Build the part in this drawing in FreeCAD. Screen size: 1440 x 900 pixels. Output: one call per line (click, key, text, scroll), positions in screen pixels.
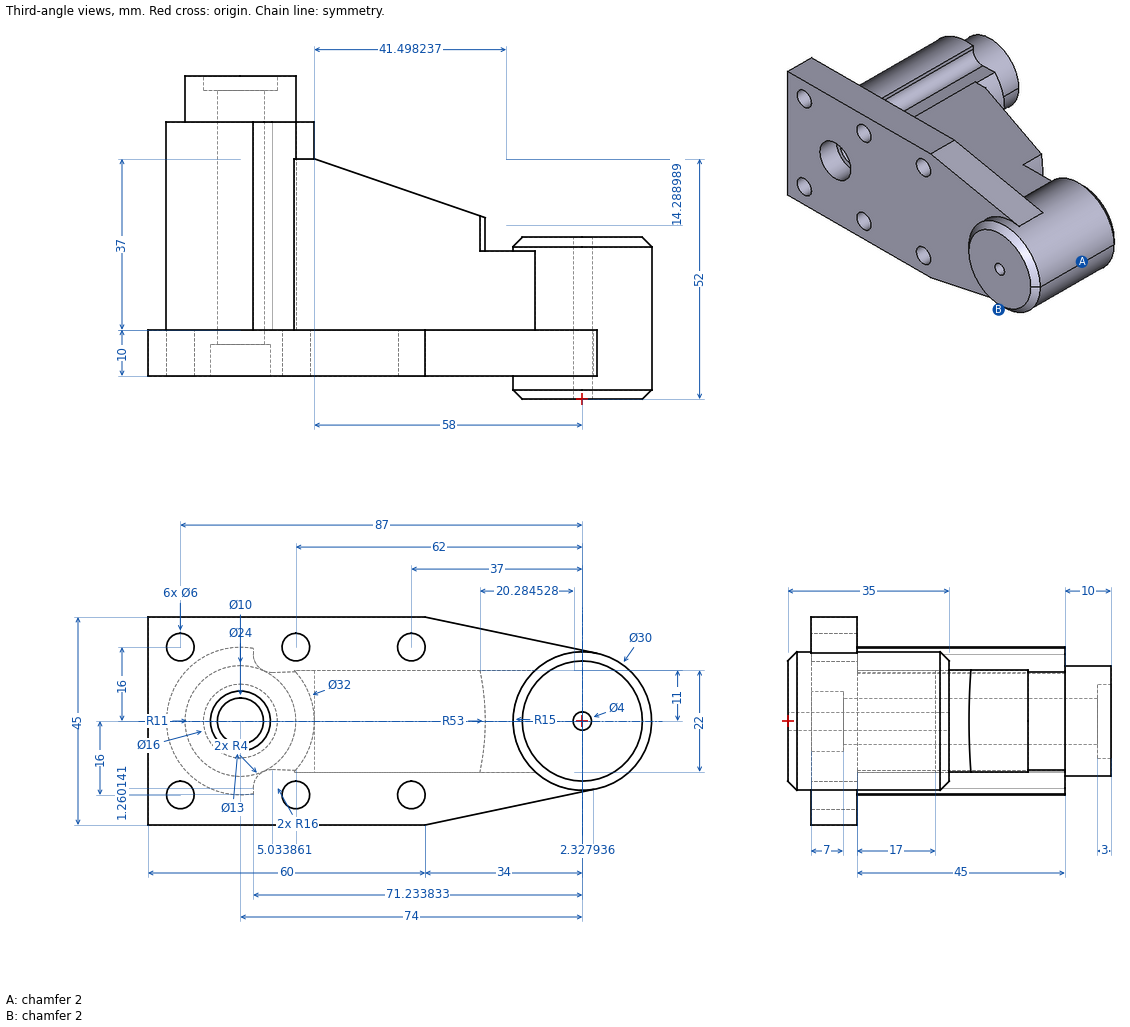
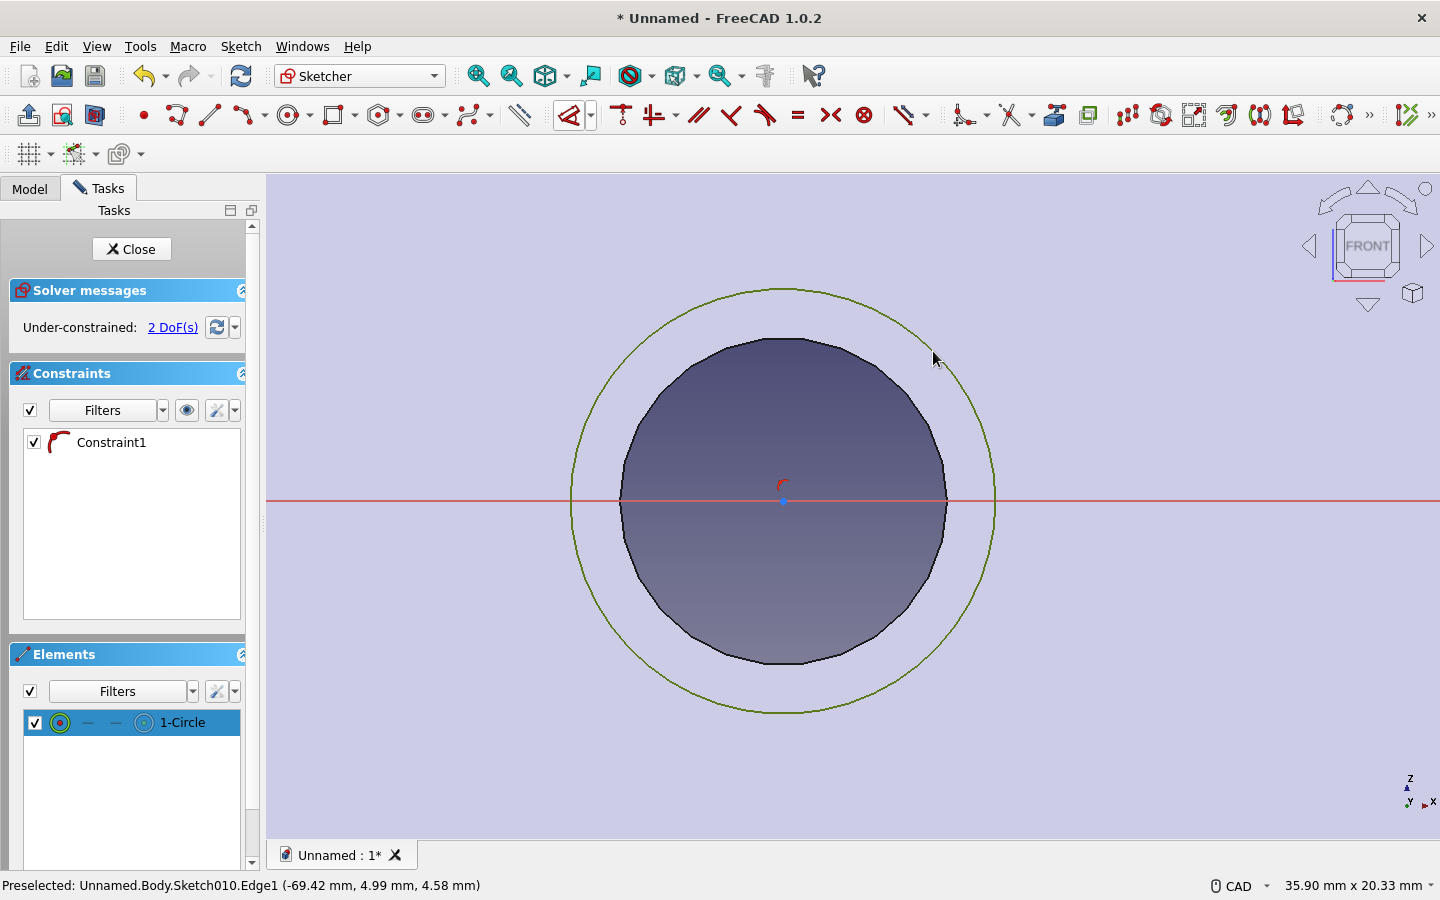
key(k)
key(o)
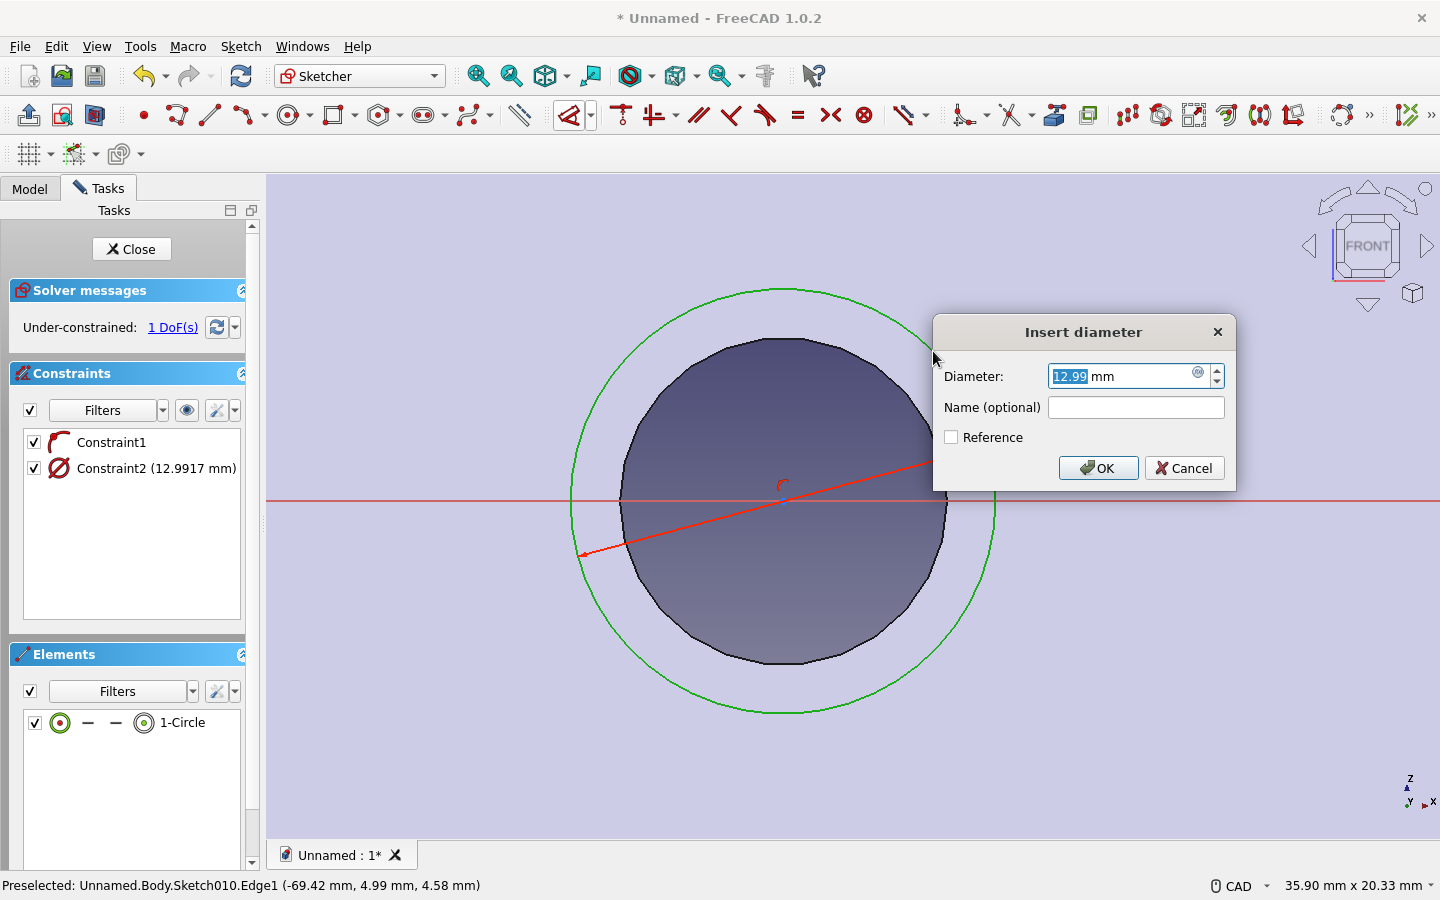
text(13)
key(Return)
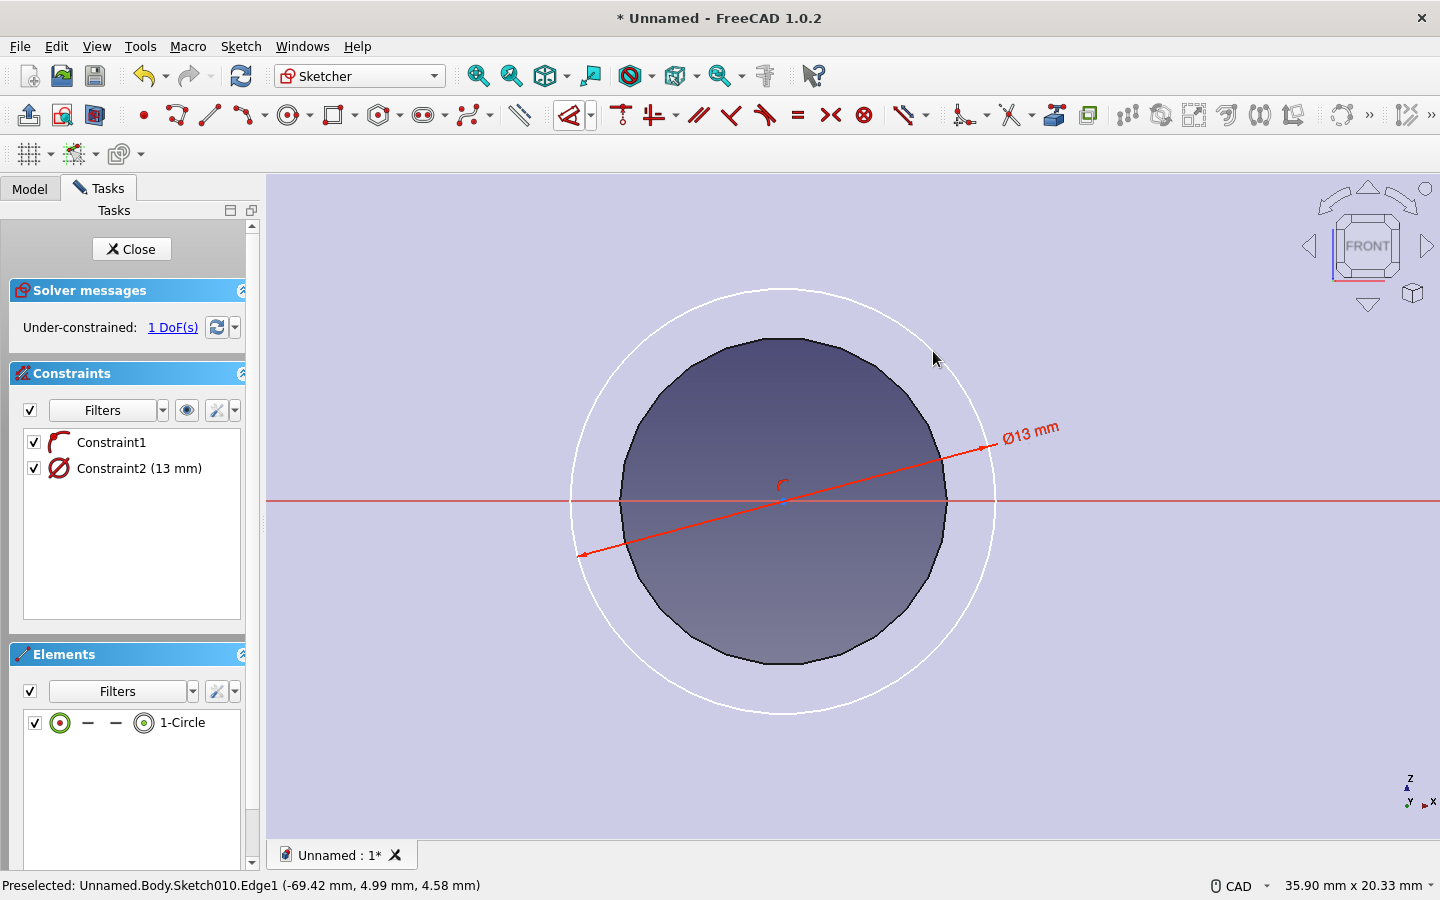
click(783, 501)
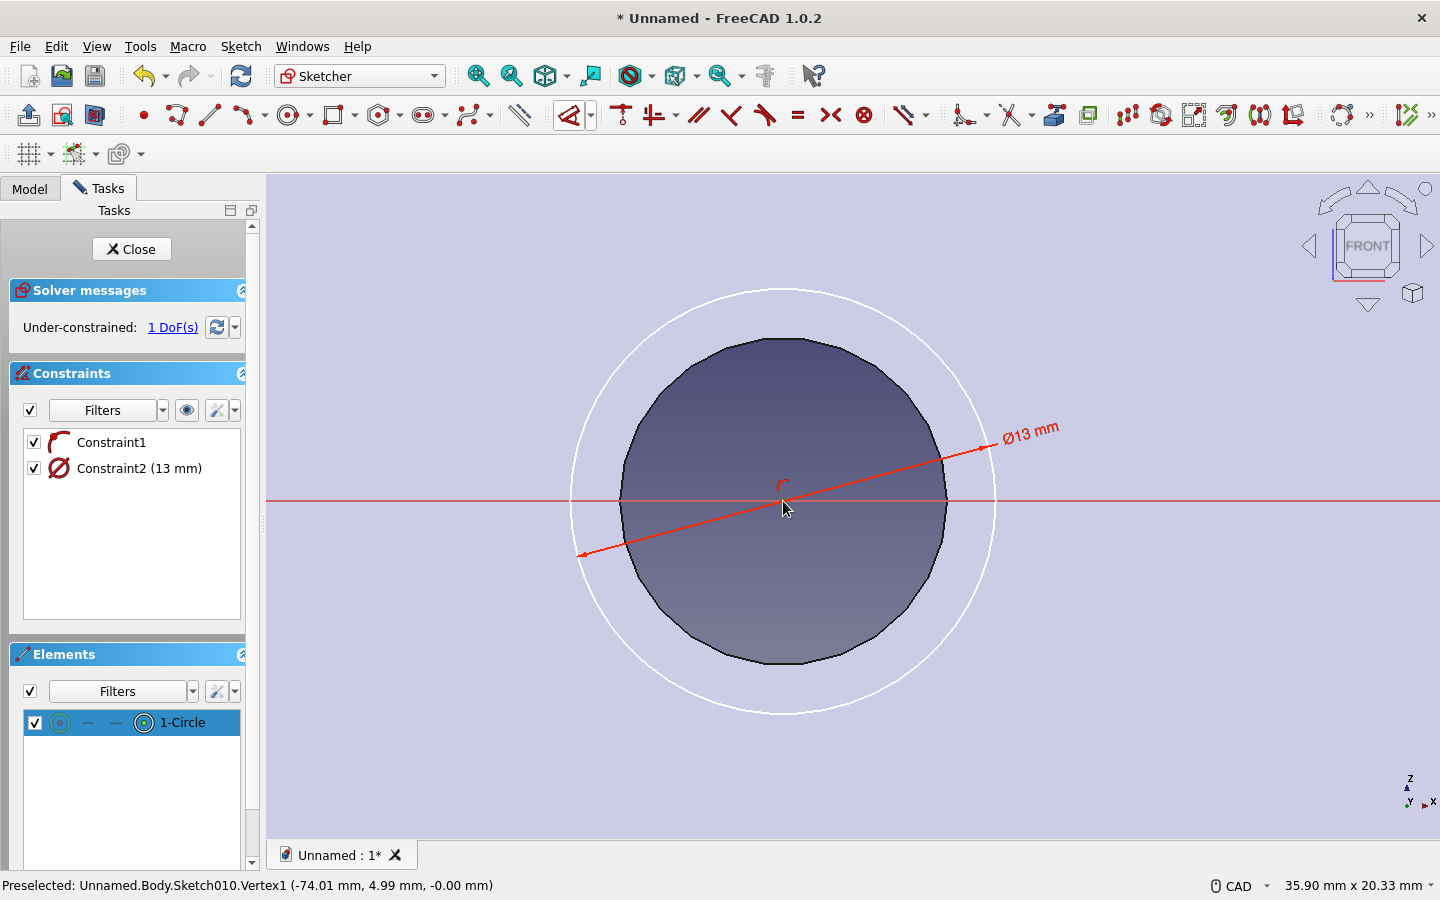
click(590, 116)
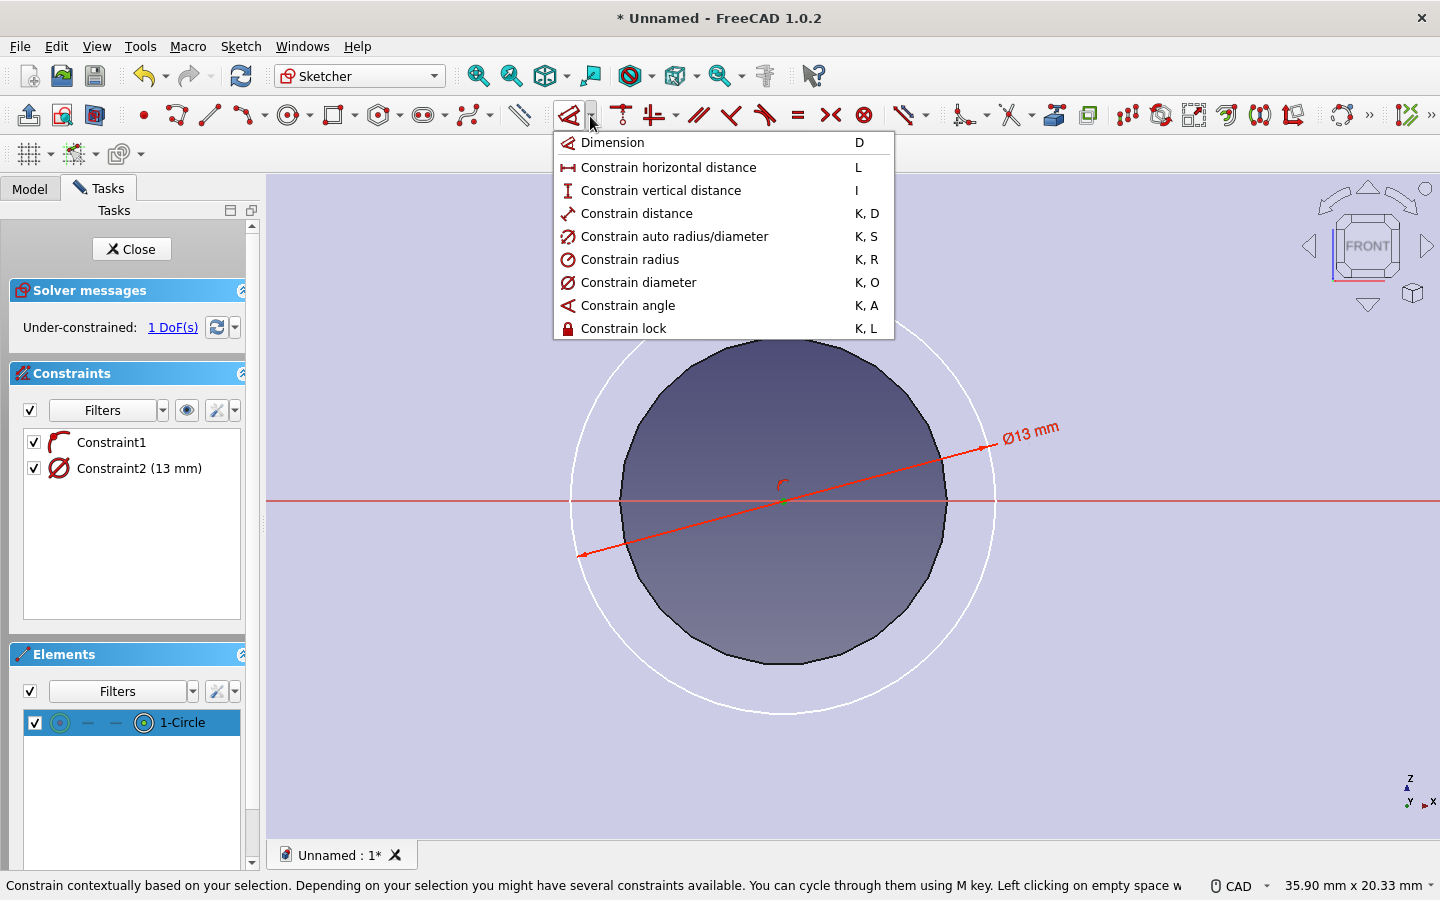
click(724, 168)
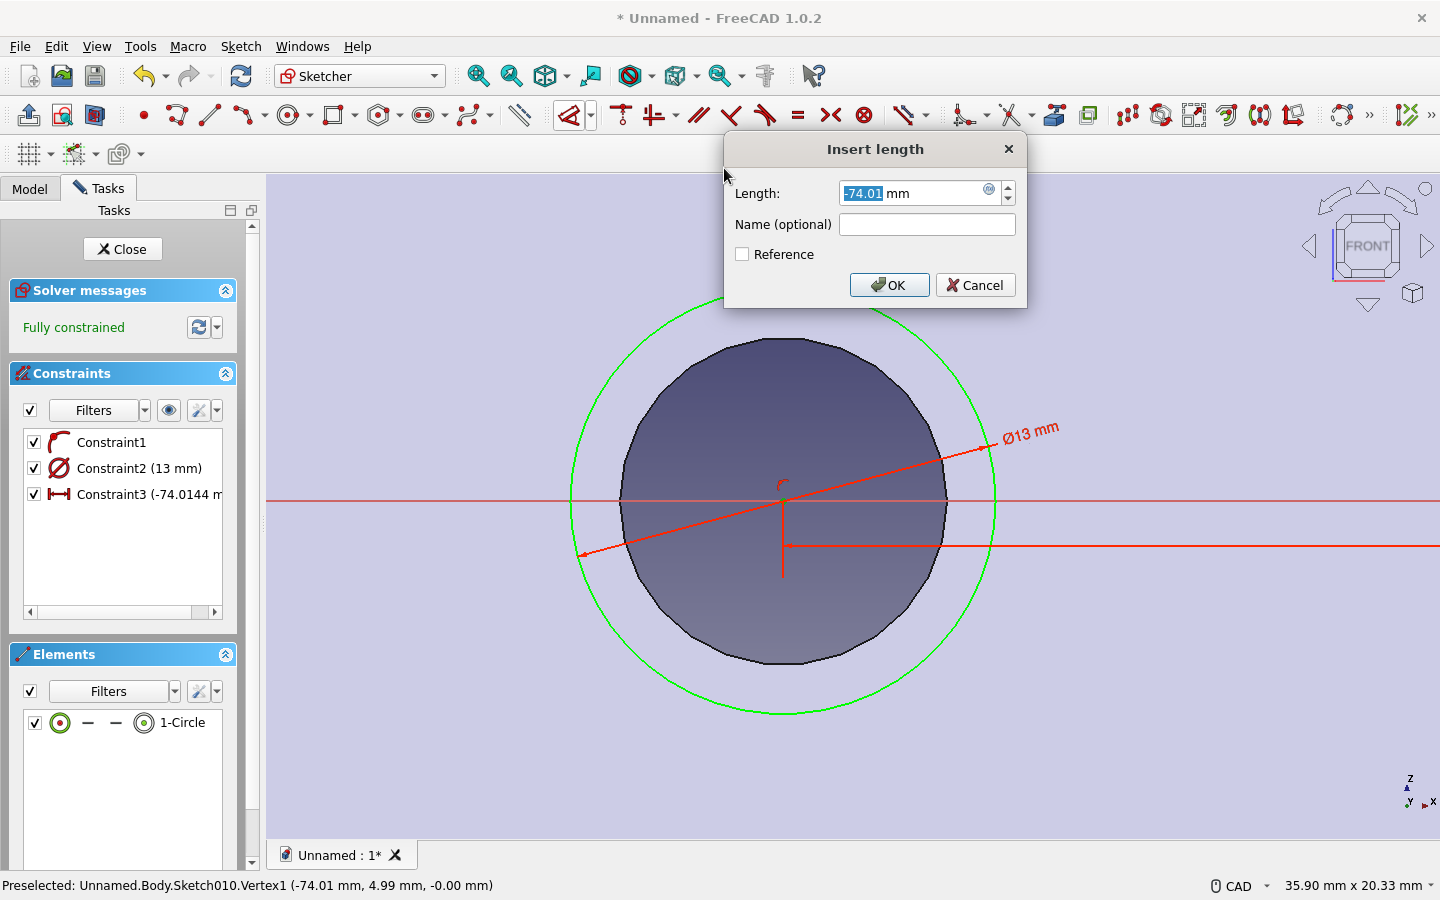
text(-74)
key(Return)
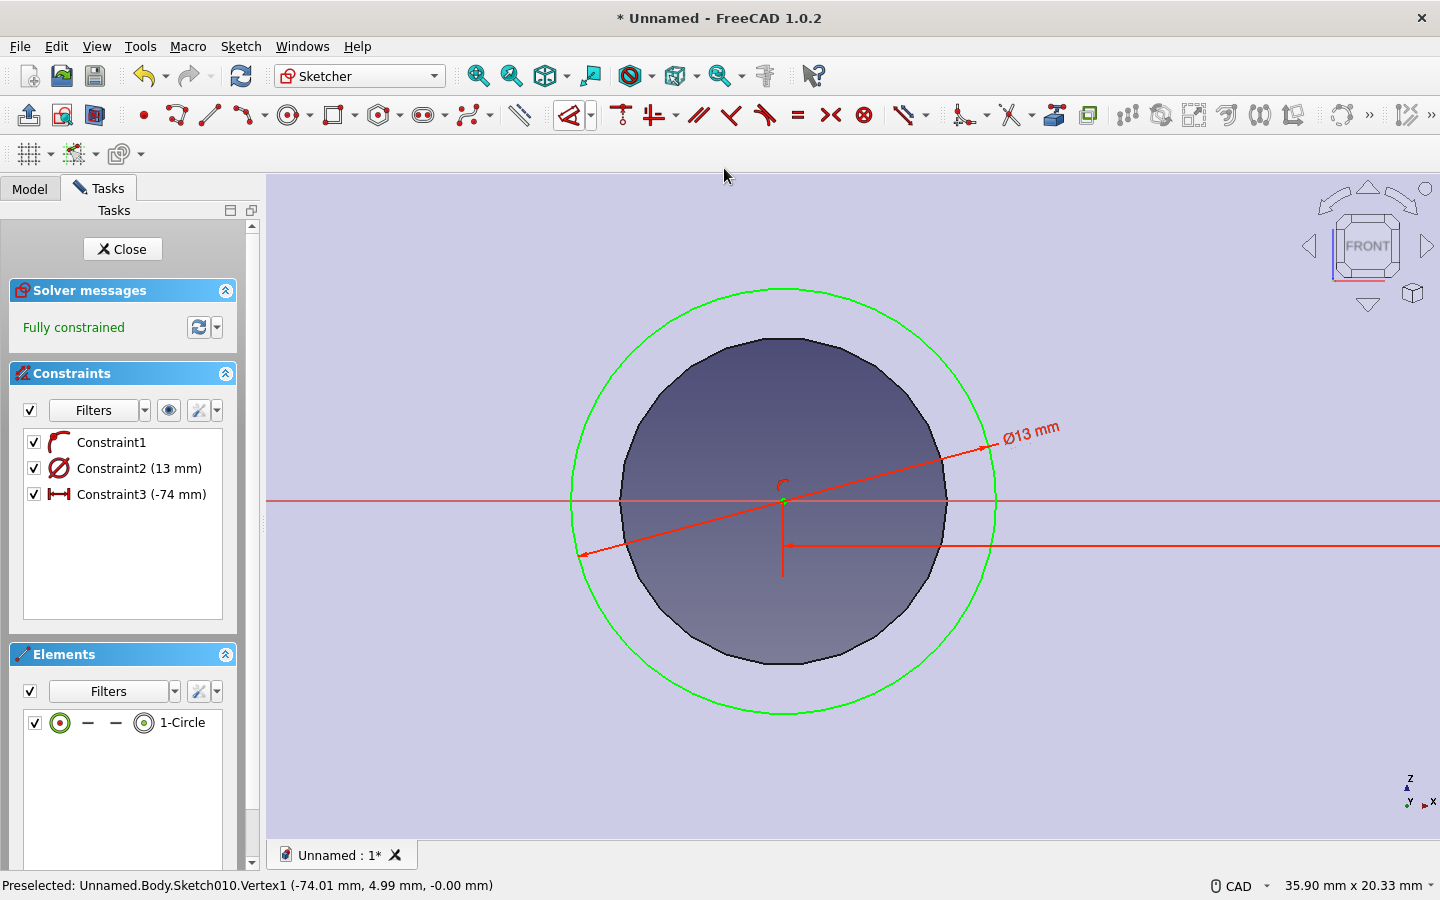
click(123, 249)